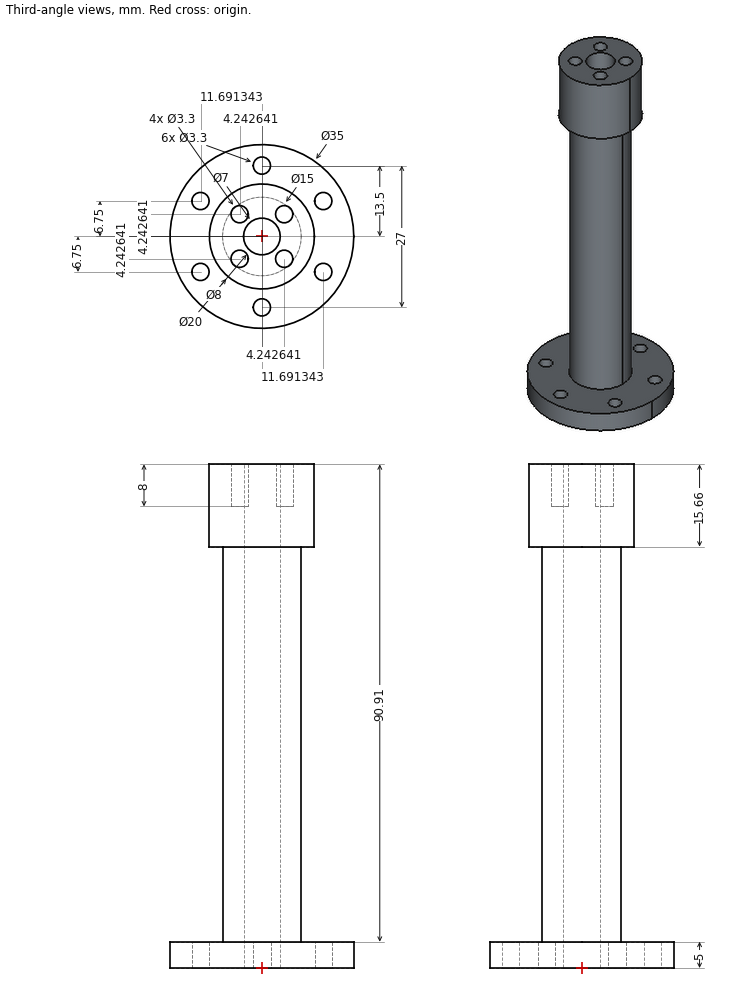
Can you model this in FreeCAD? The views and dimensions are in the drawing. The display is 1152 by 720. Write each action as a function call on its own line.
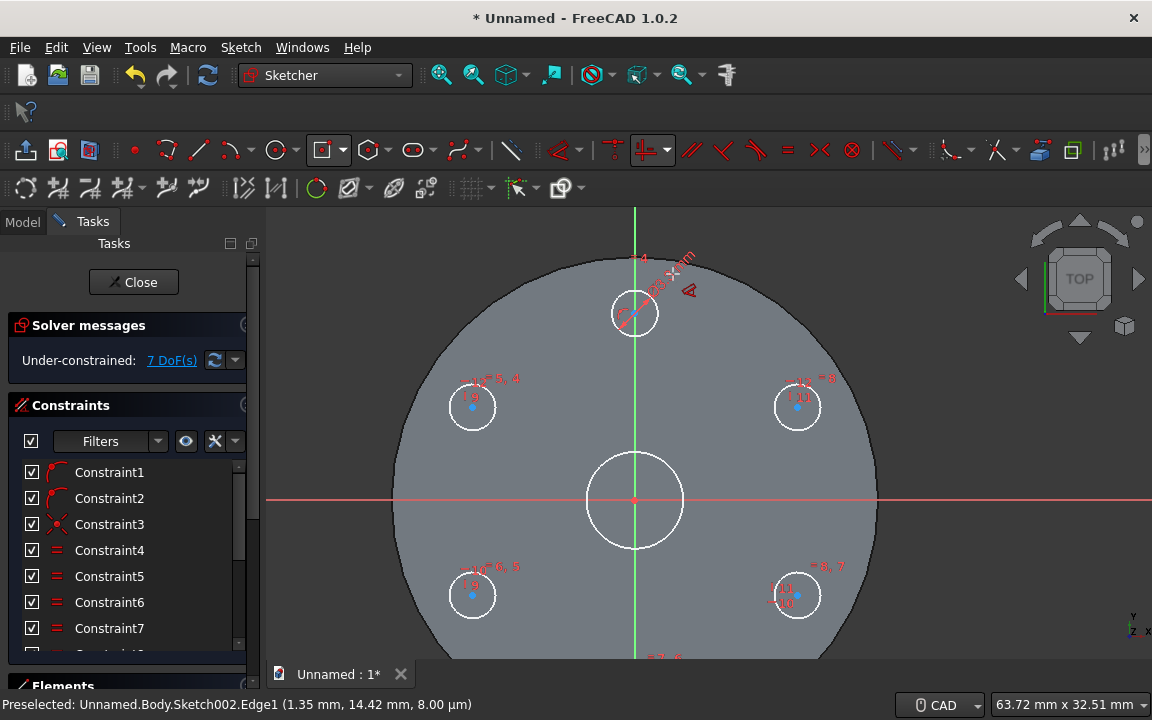
click(669, 466)
click(692, 443)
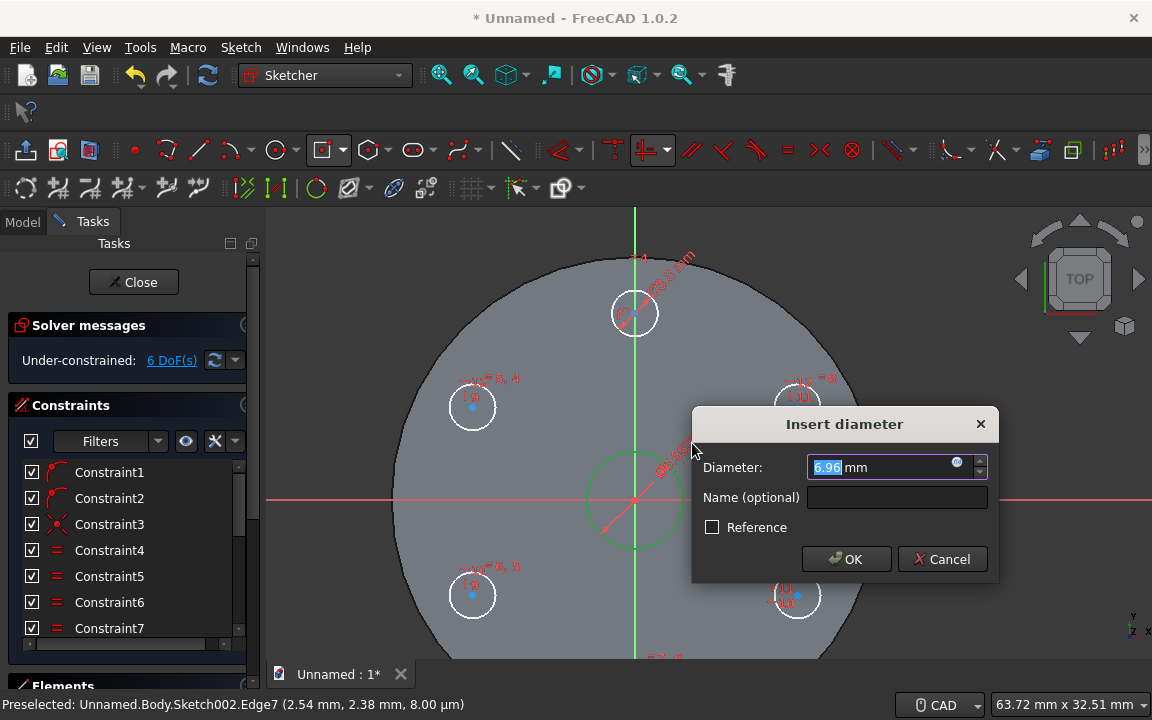
text(7)
key(Return)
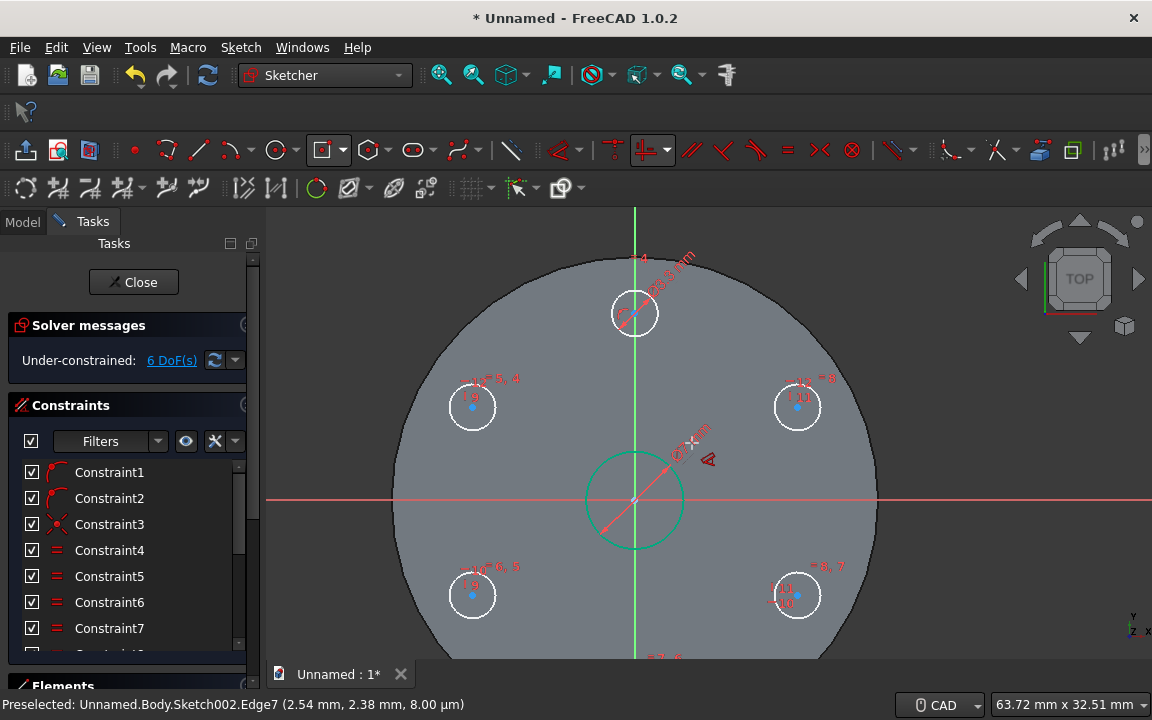
click(635, 313)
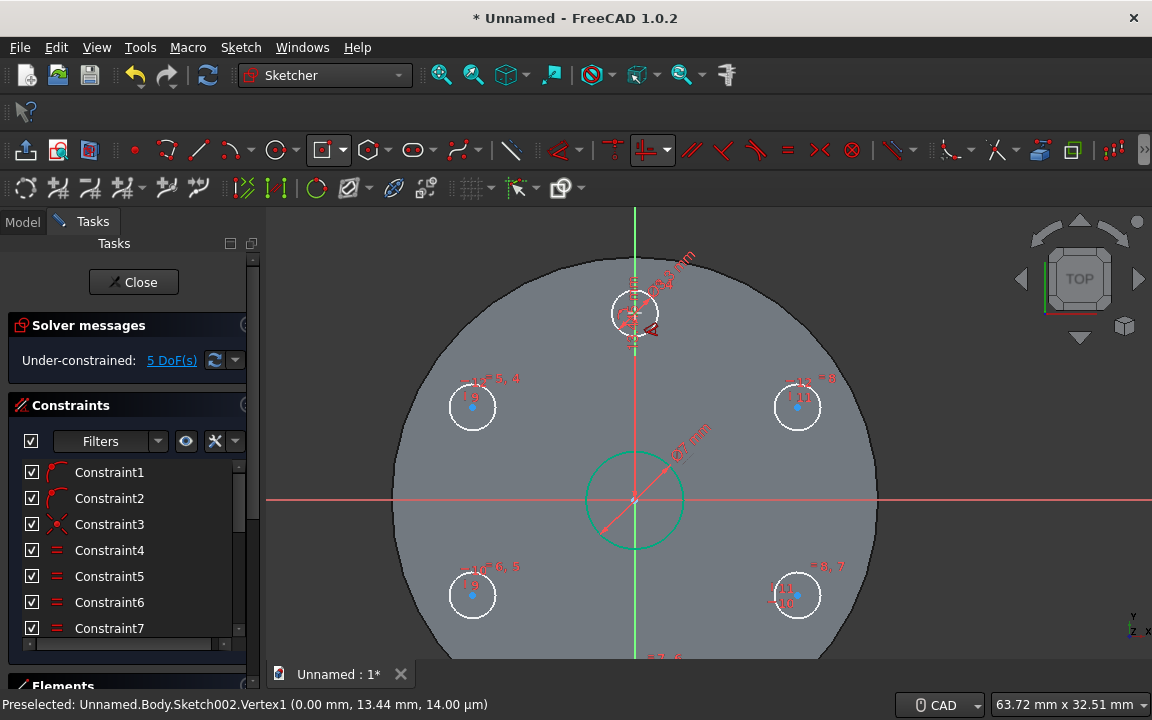
scroll(652, 296, down, 2)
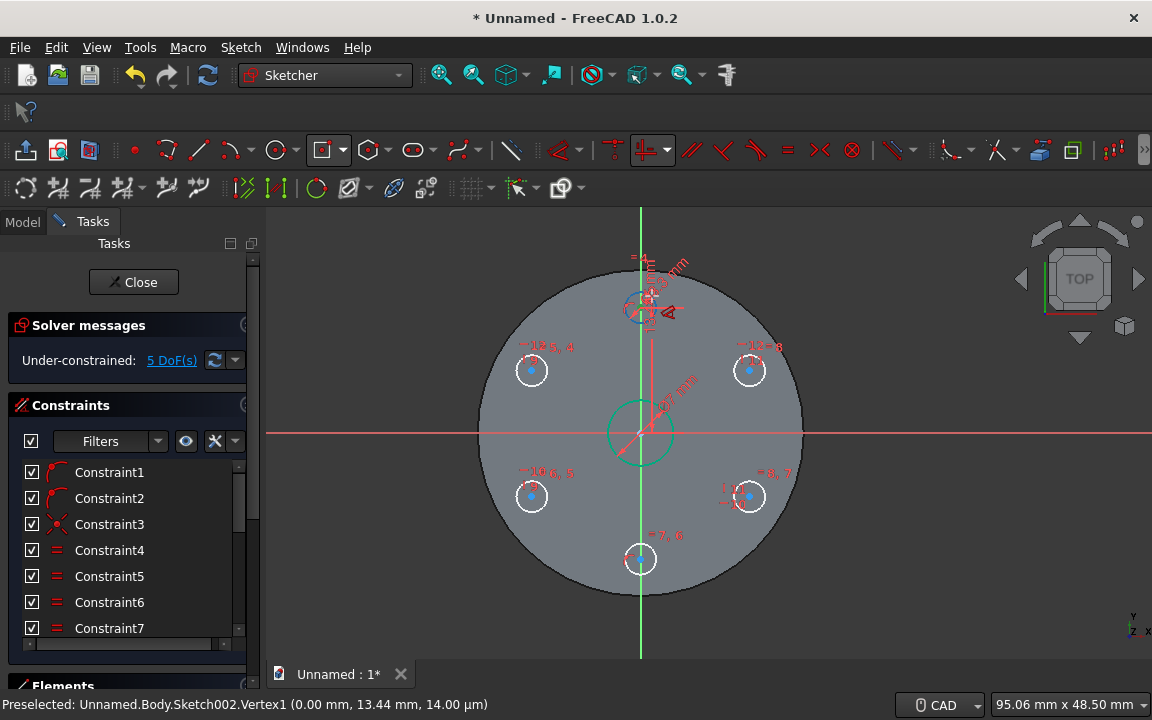
click(641, 559)
click(675, 491)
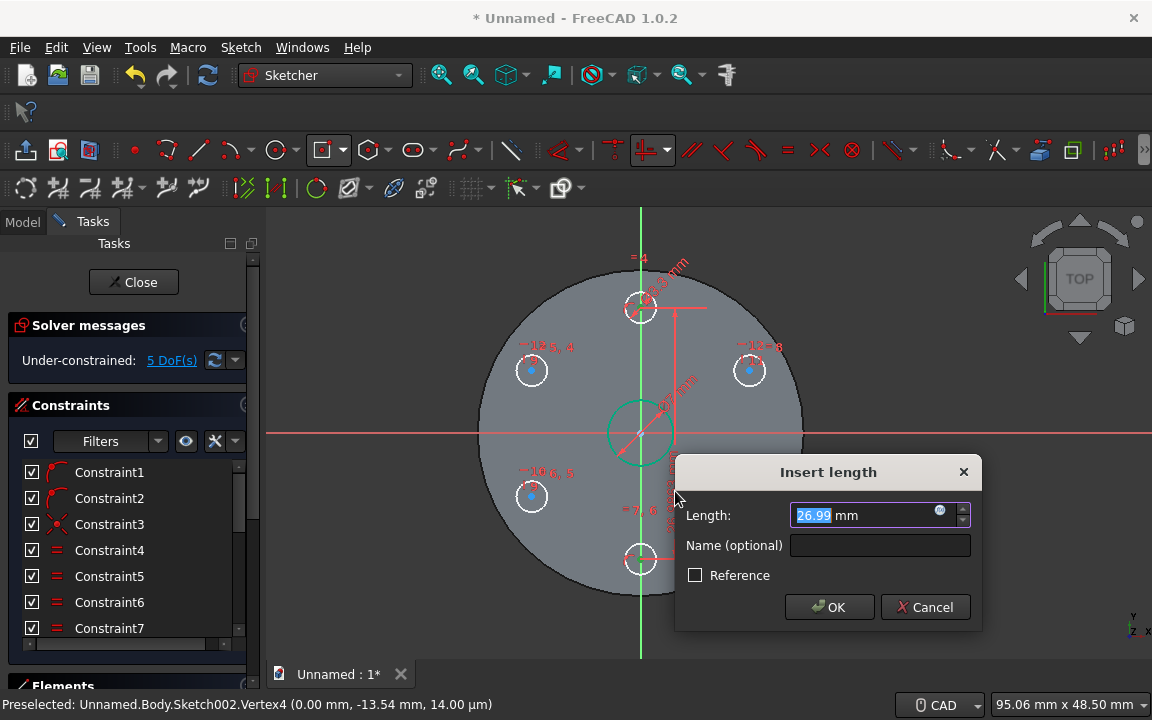
text(27)
key(Return)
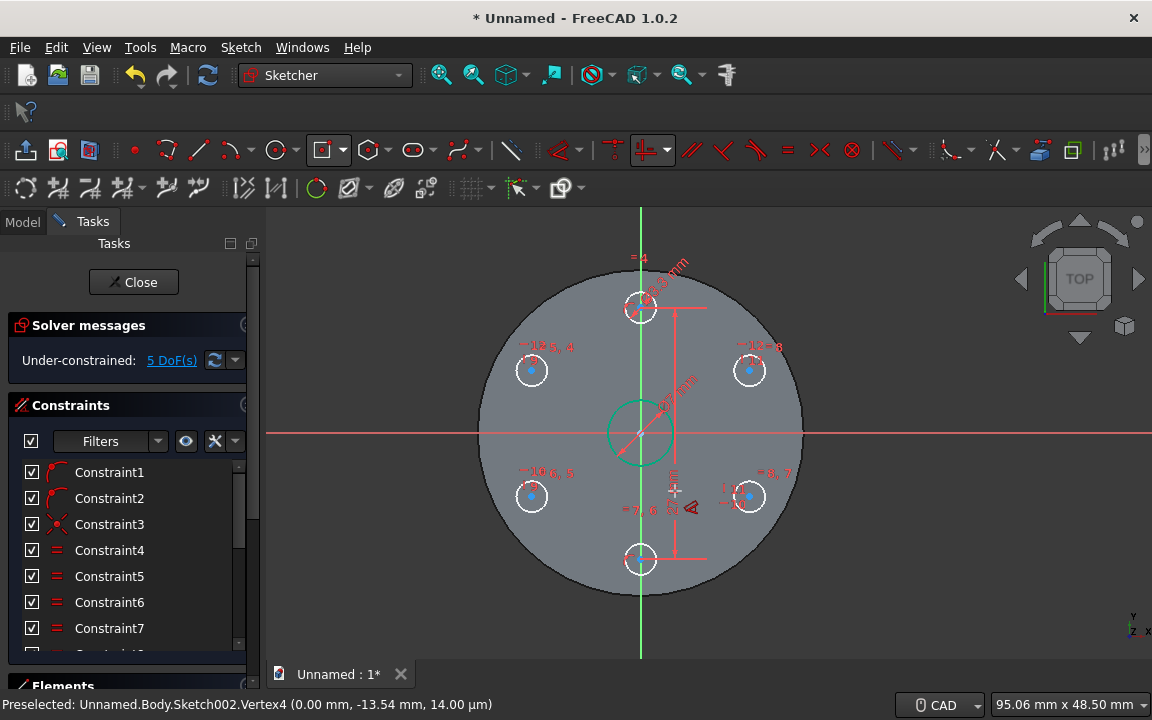
click(641, 308)
click(675, 370)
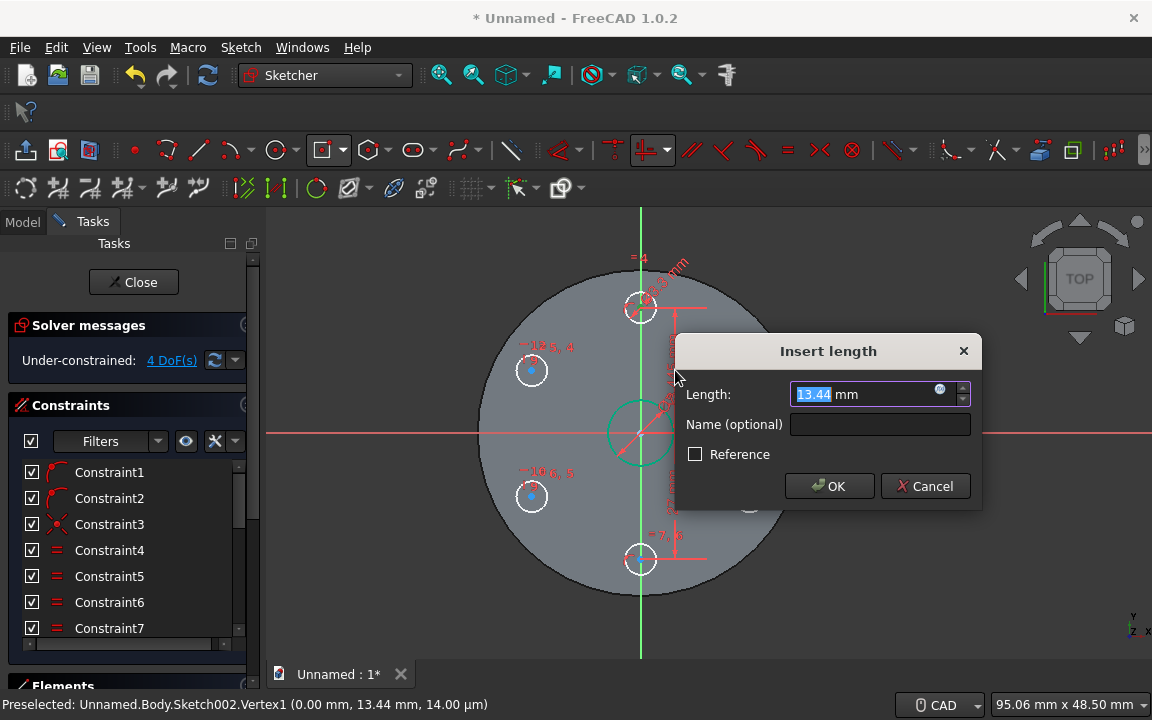
text(13.5)
key(Return)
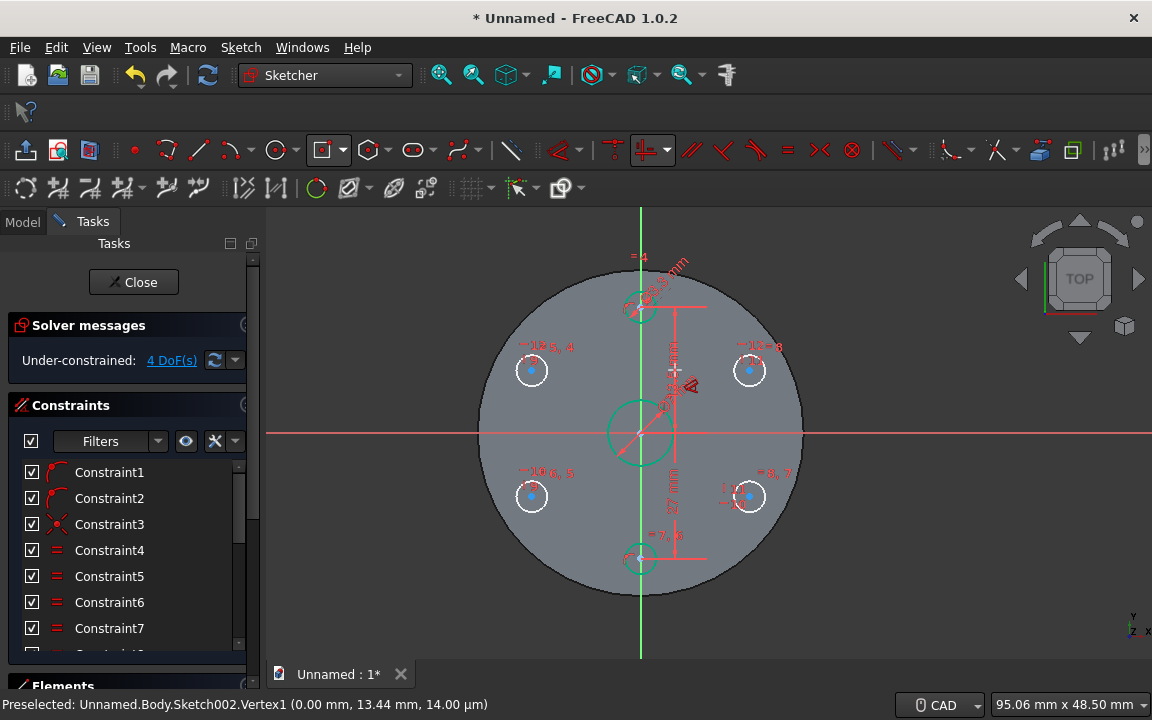
click(532, 371)
click(498, 402)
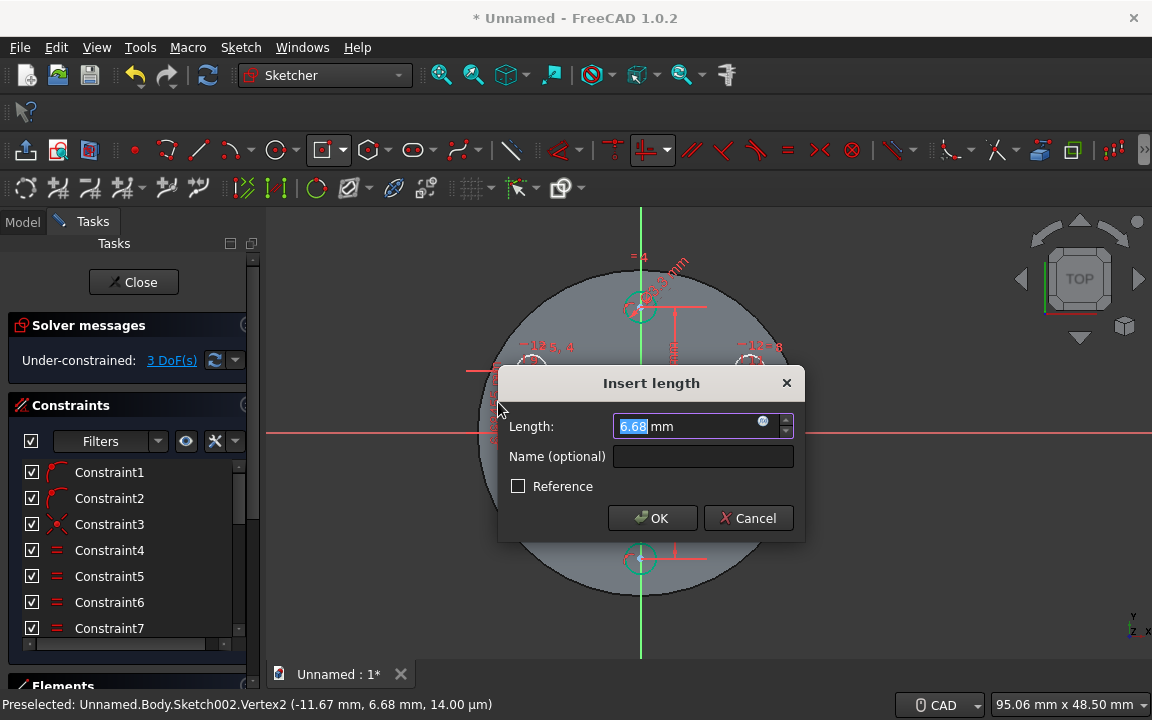
text(6.75)
key(Return)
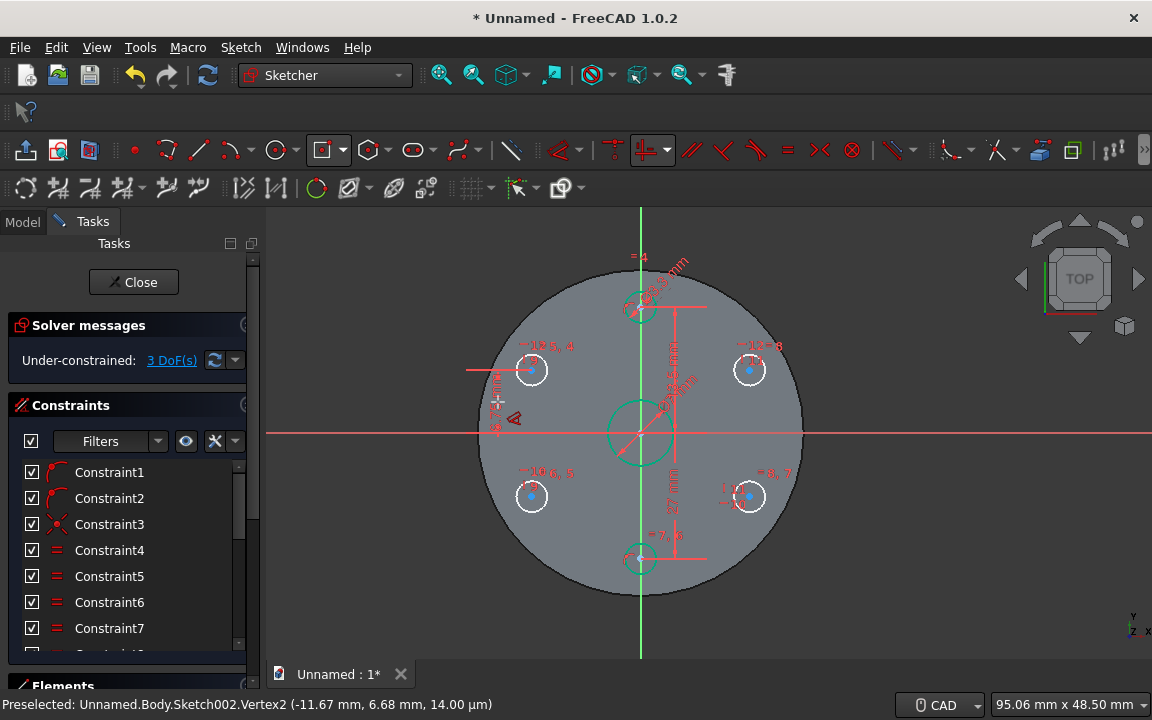
click(532, 497)
click(498, 465)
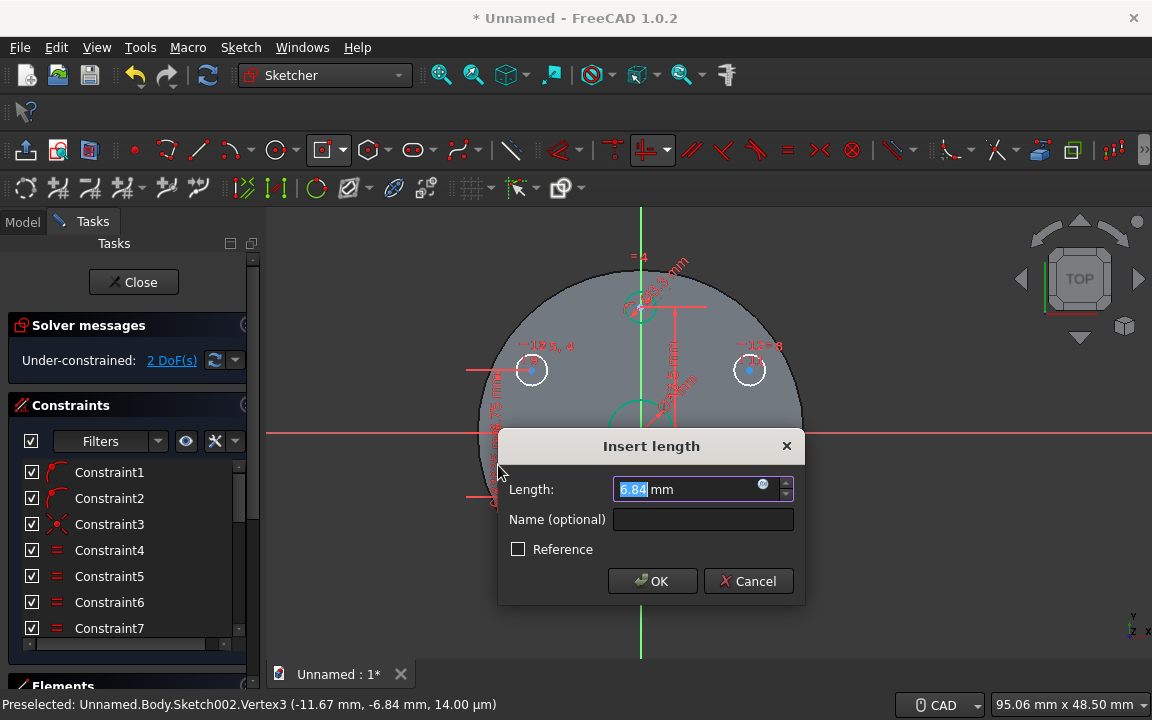
text(6.75)
key(Return)